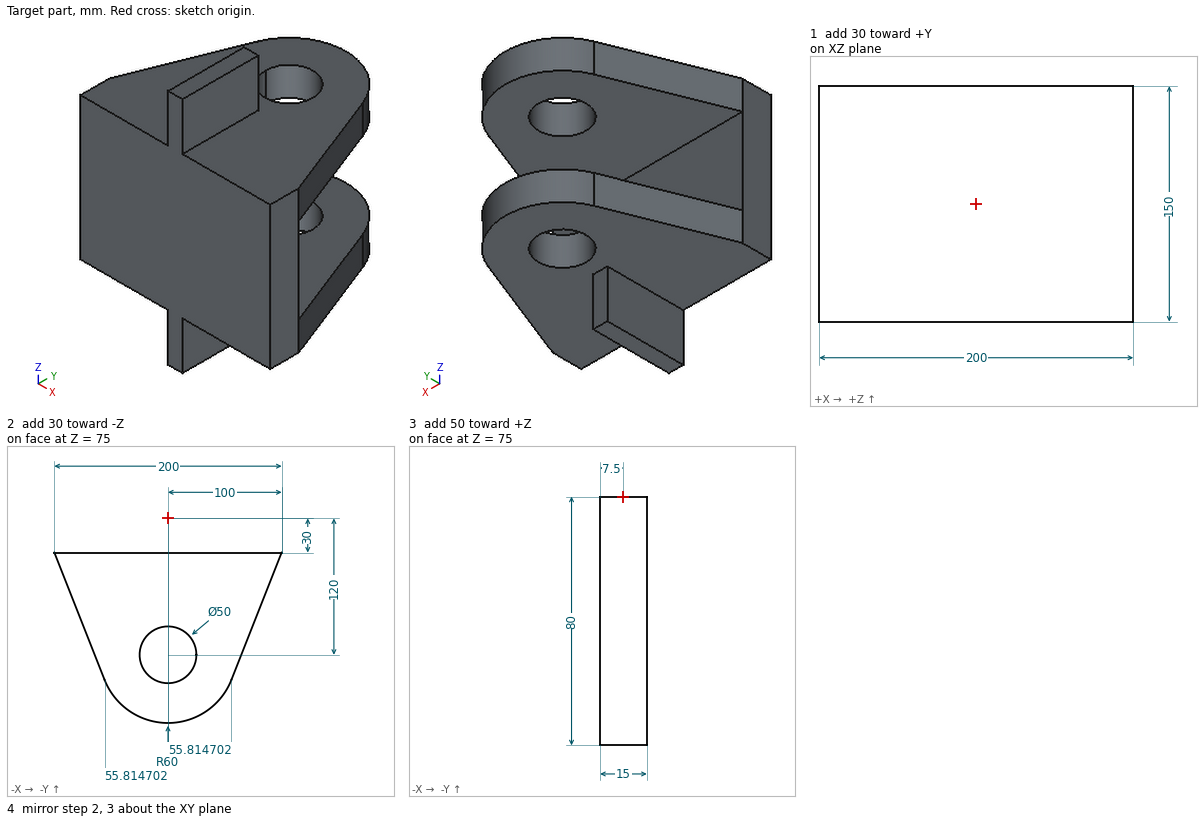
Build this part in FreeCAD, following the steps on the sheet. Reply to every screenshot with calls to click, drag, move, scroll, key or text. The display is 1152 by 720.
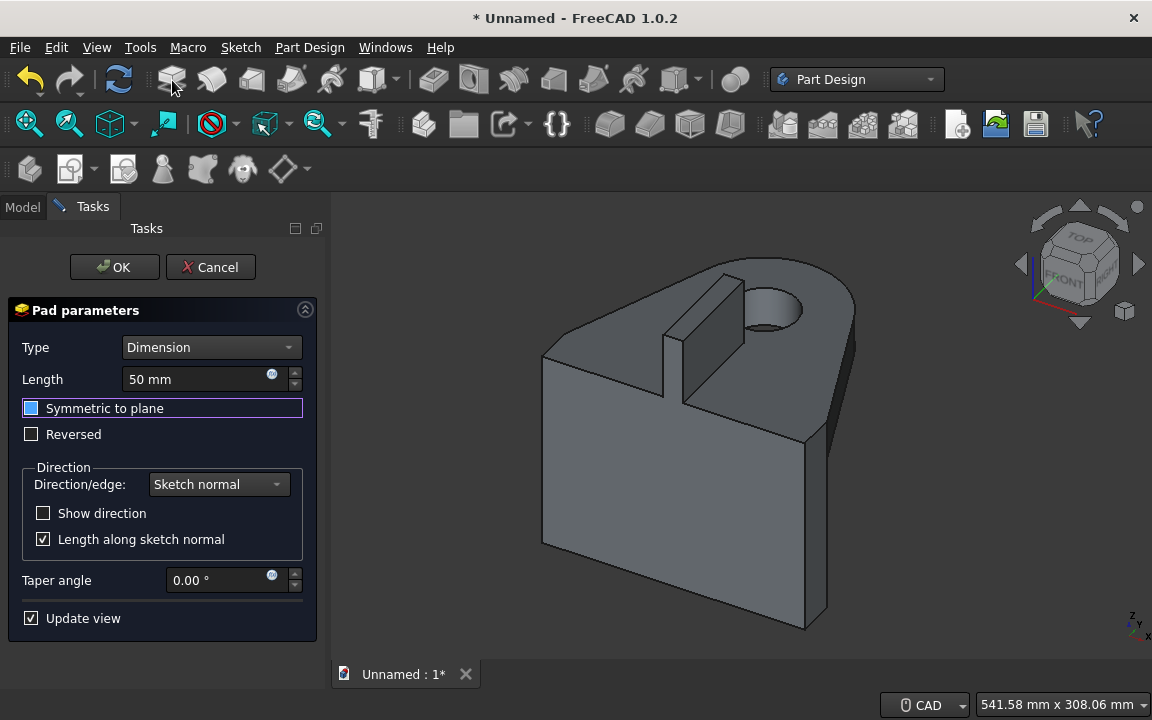
click(115, 267)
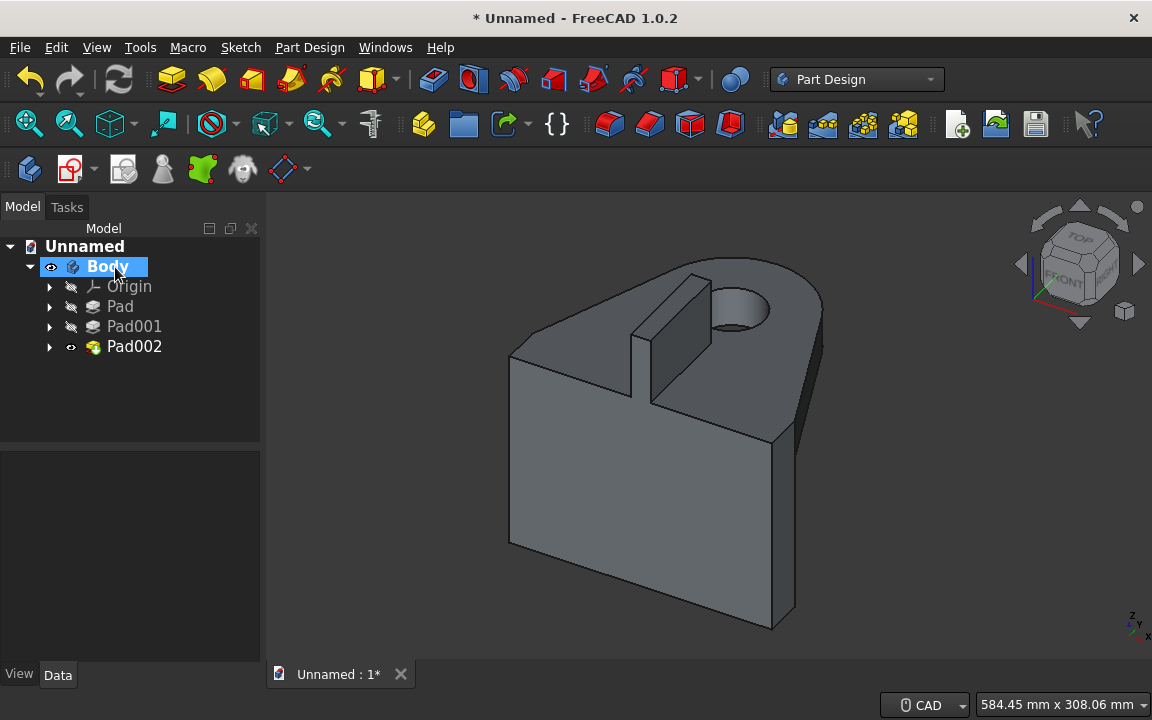
key(v)
key(f)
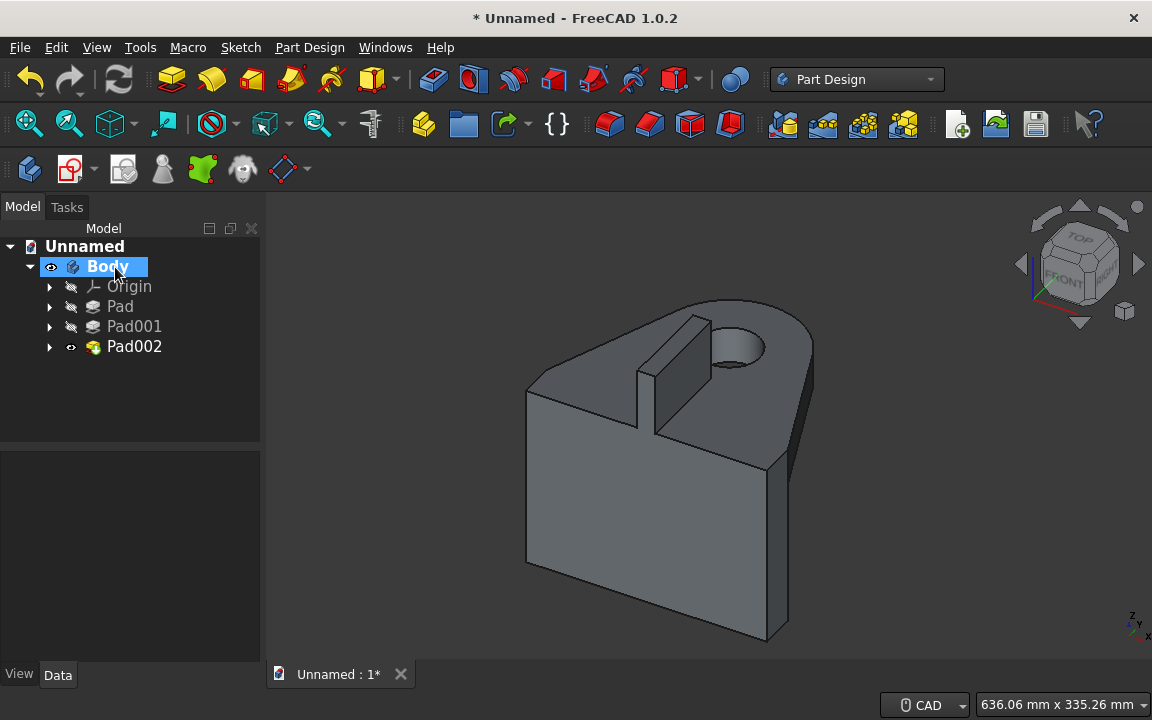
click(116, 327)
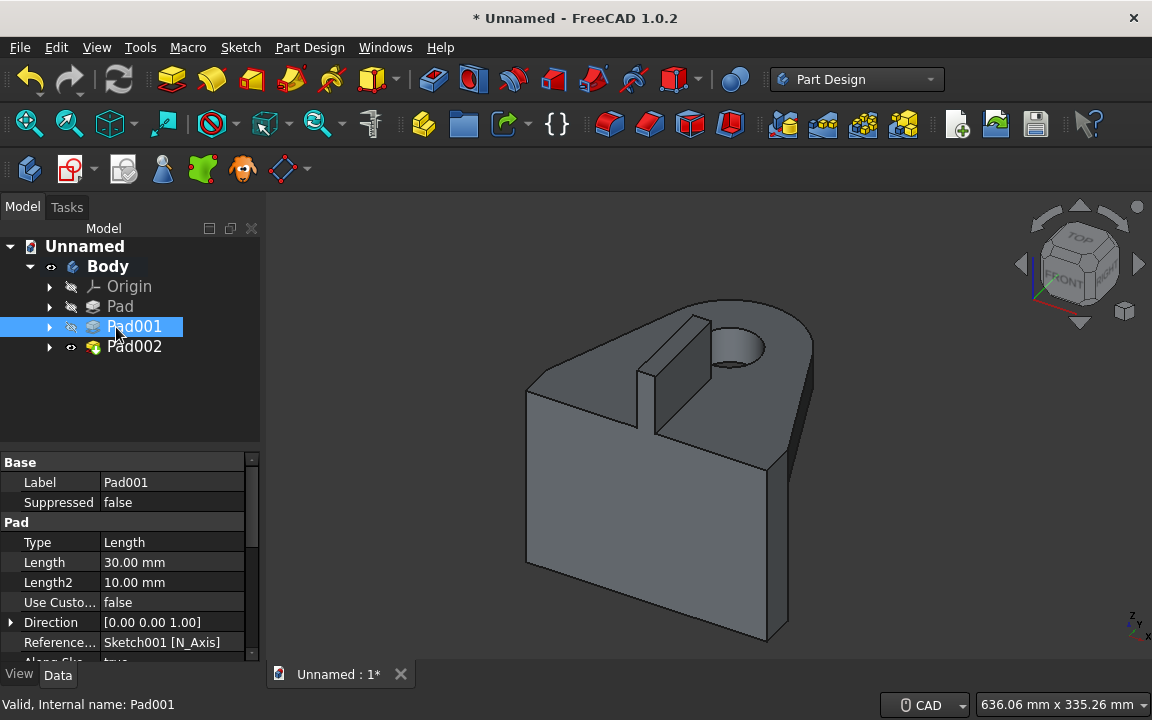
click(116, 347, ctrl)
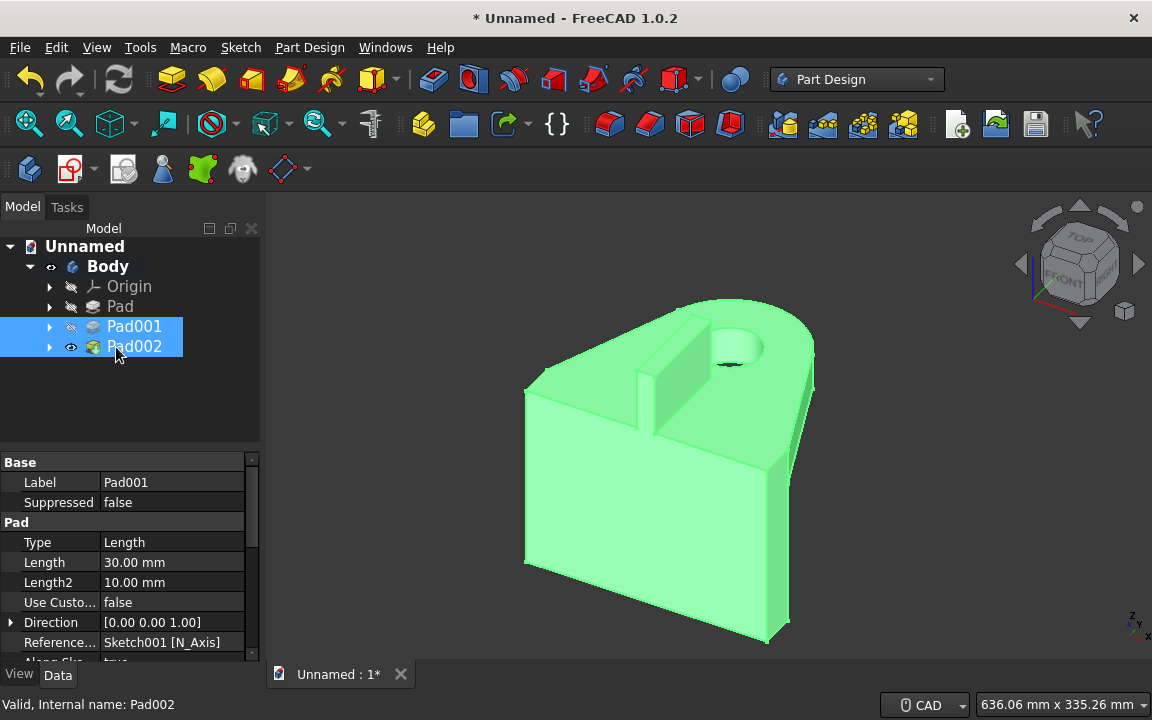
click(784, 124)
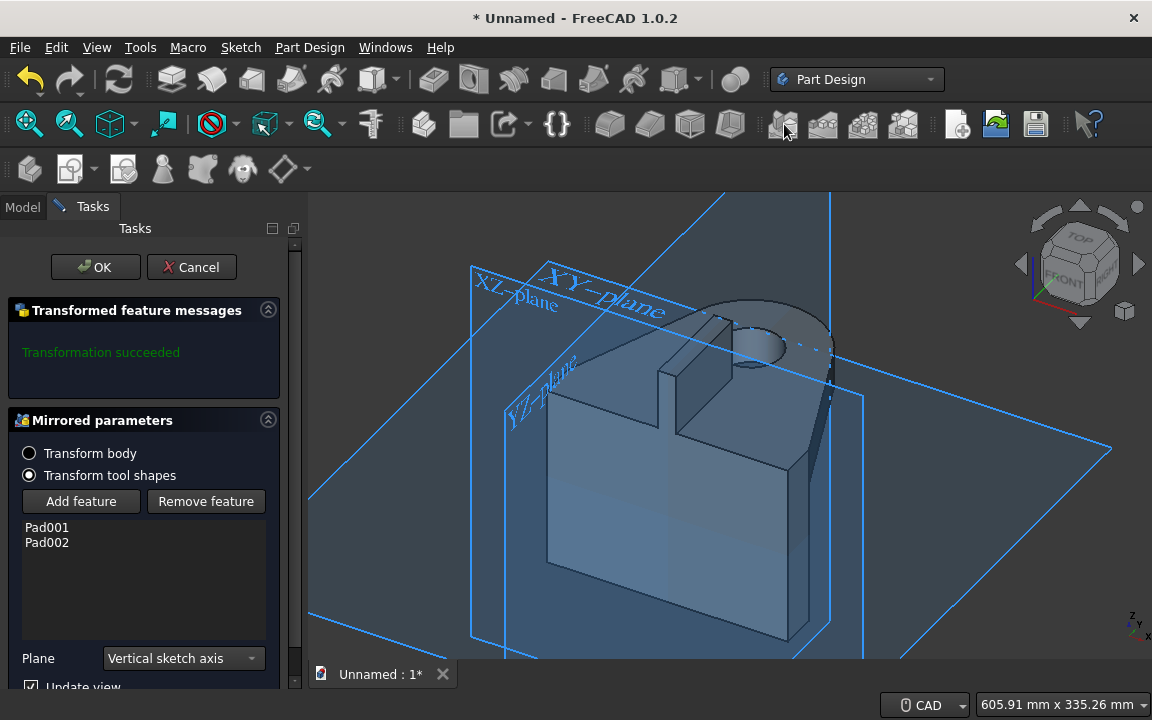
click(184, 658)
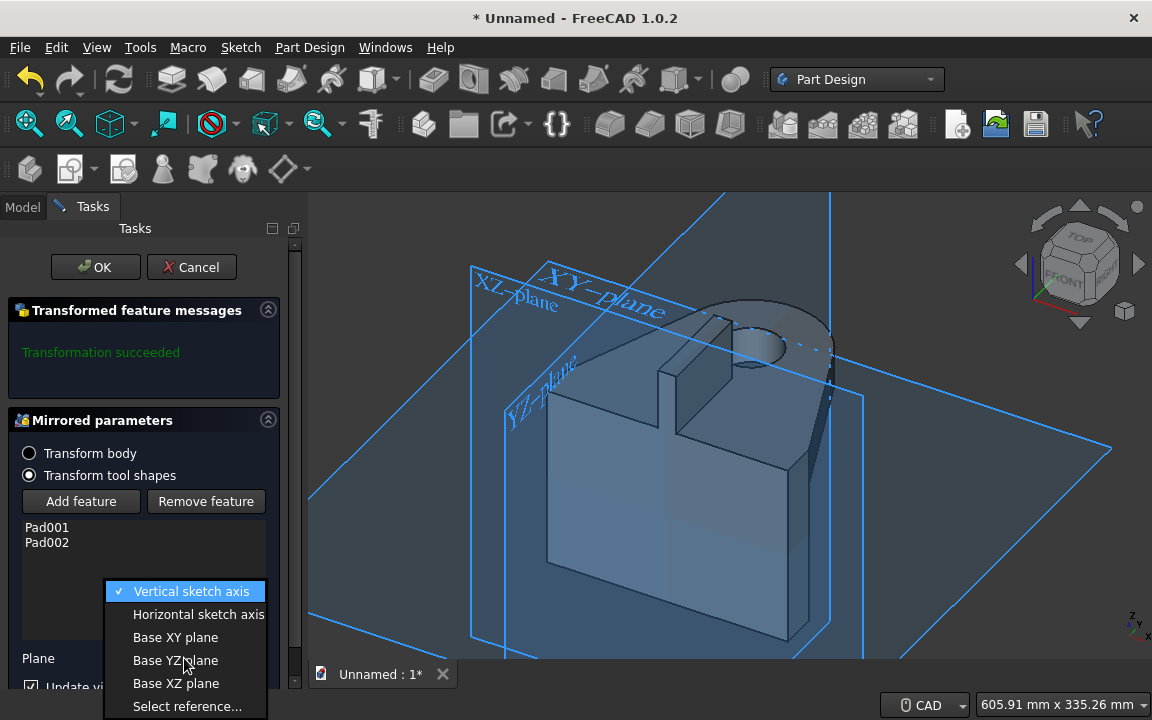
click(184, 638)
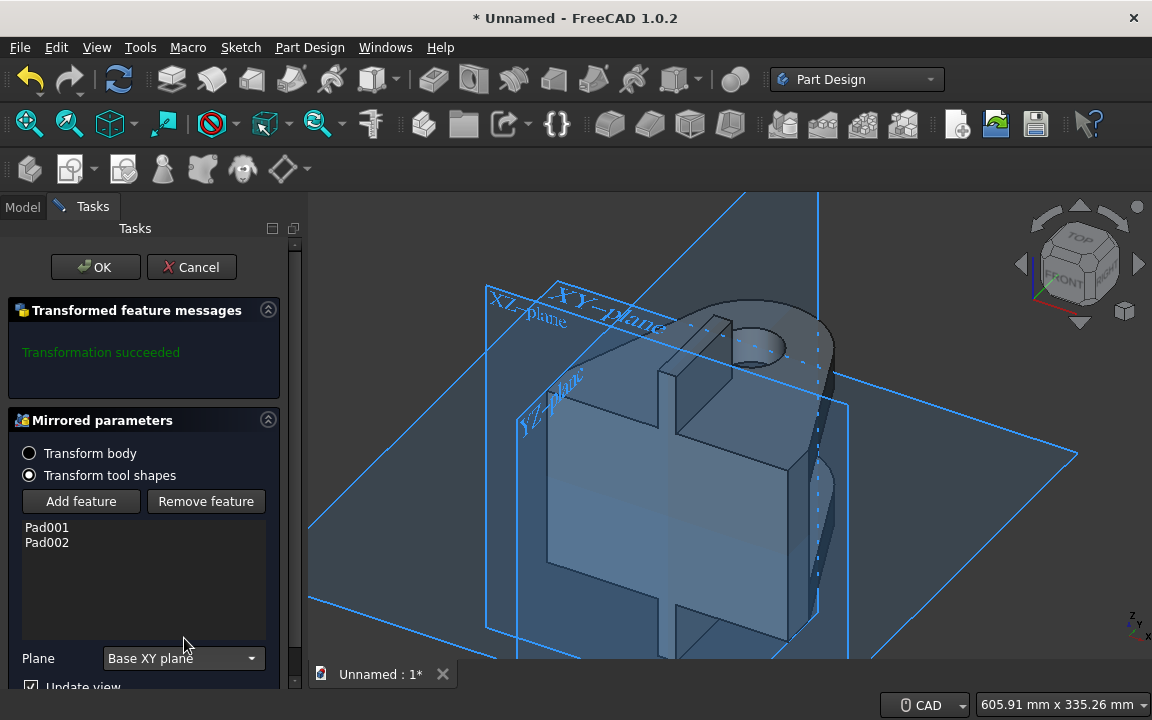
click(96, 267)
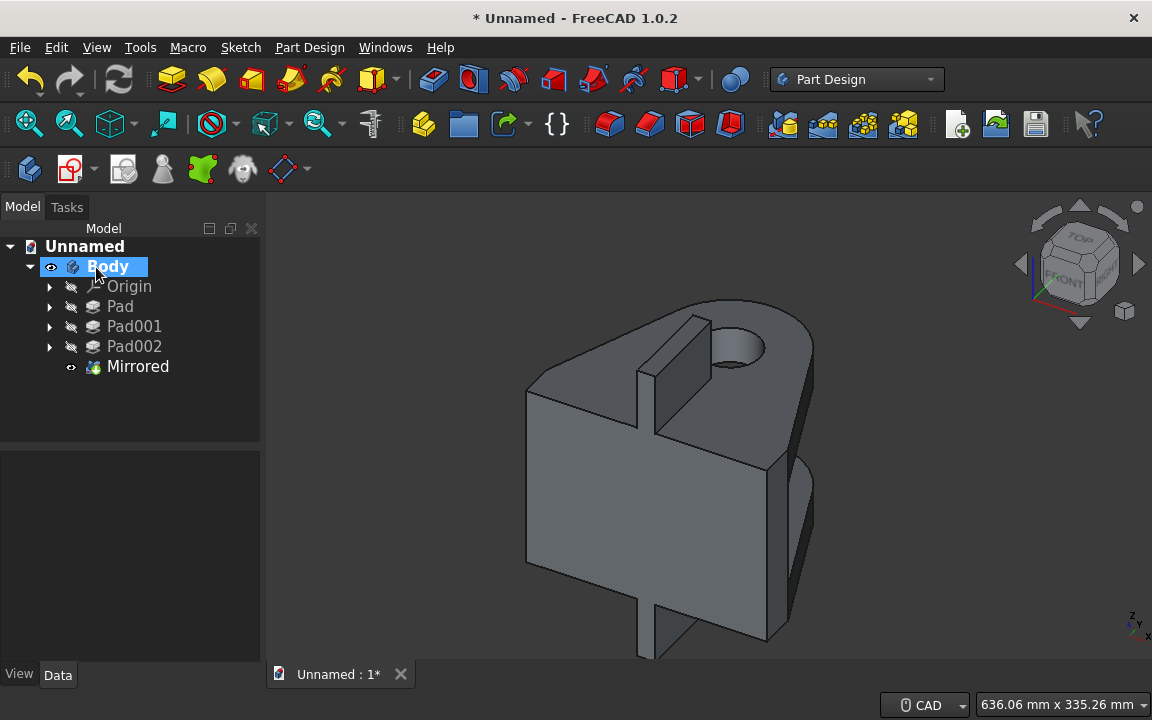
key(0)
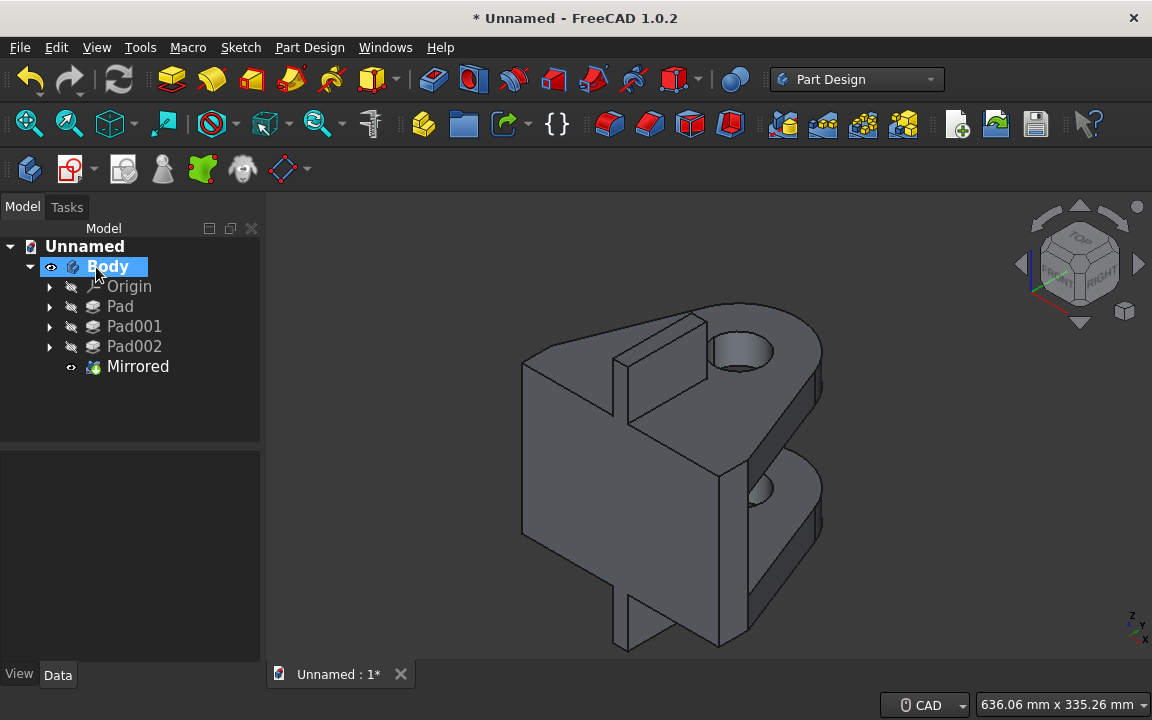
click(30, 124)